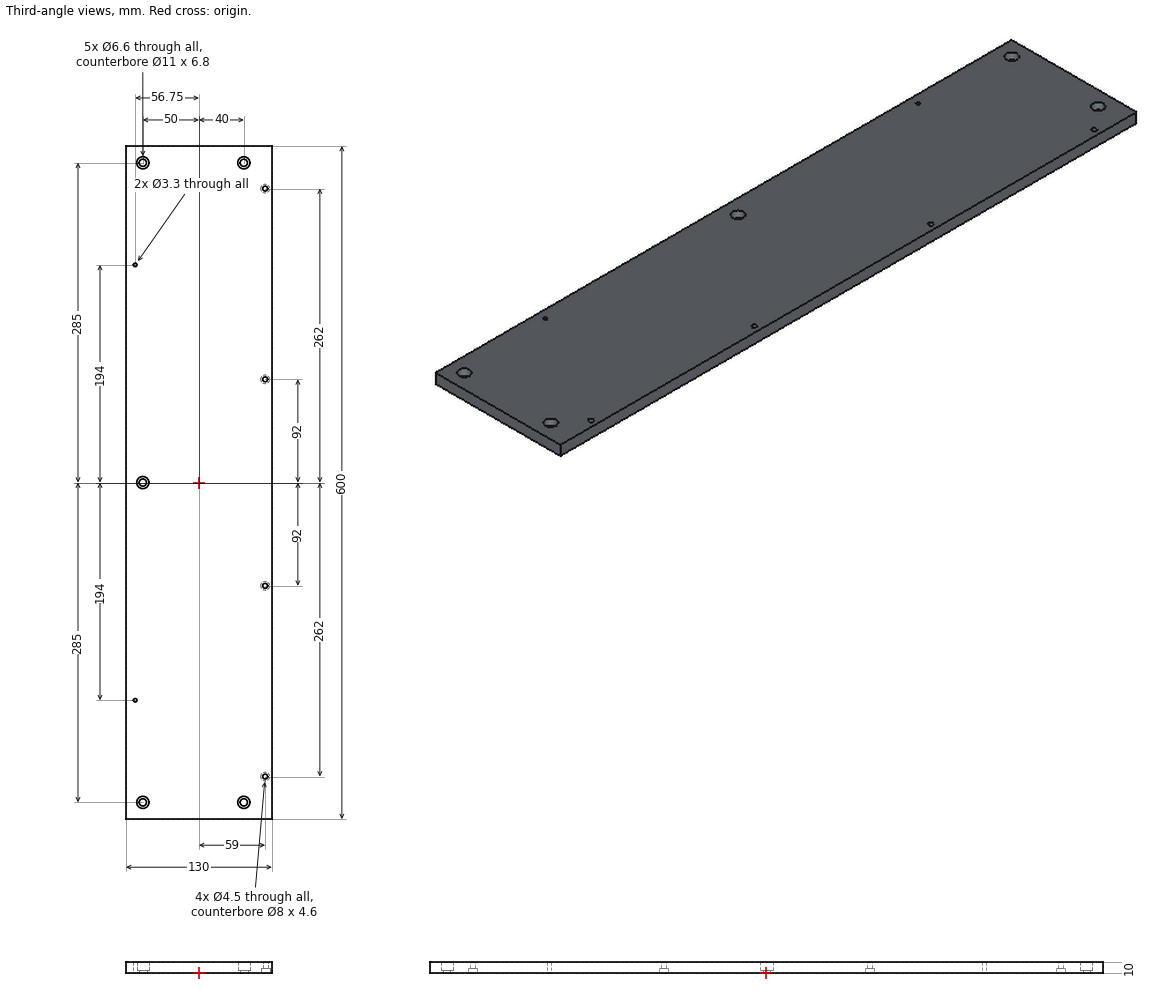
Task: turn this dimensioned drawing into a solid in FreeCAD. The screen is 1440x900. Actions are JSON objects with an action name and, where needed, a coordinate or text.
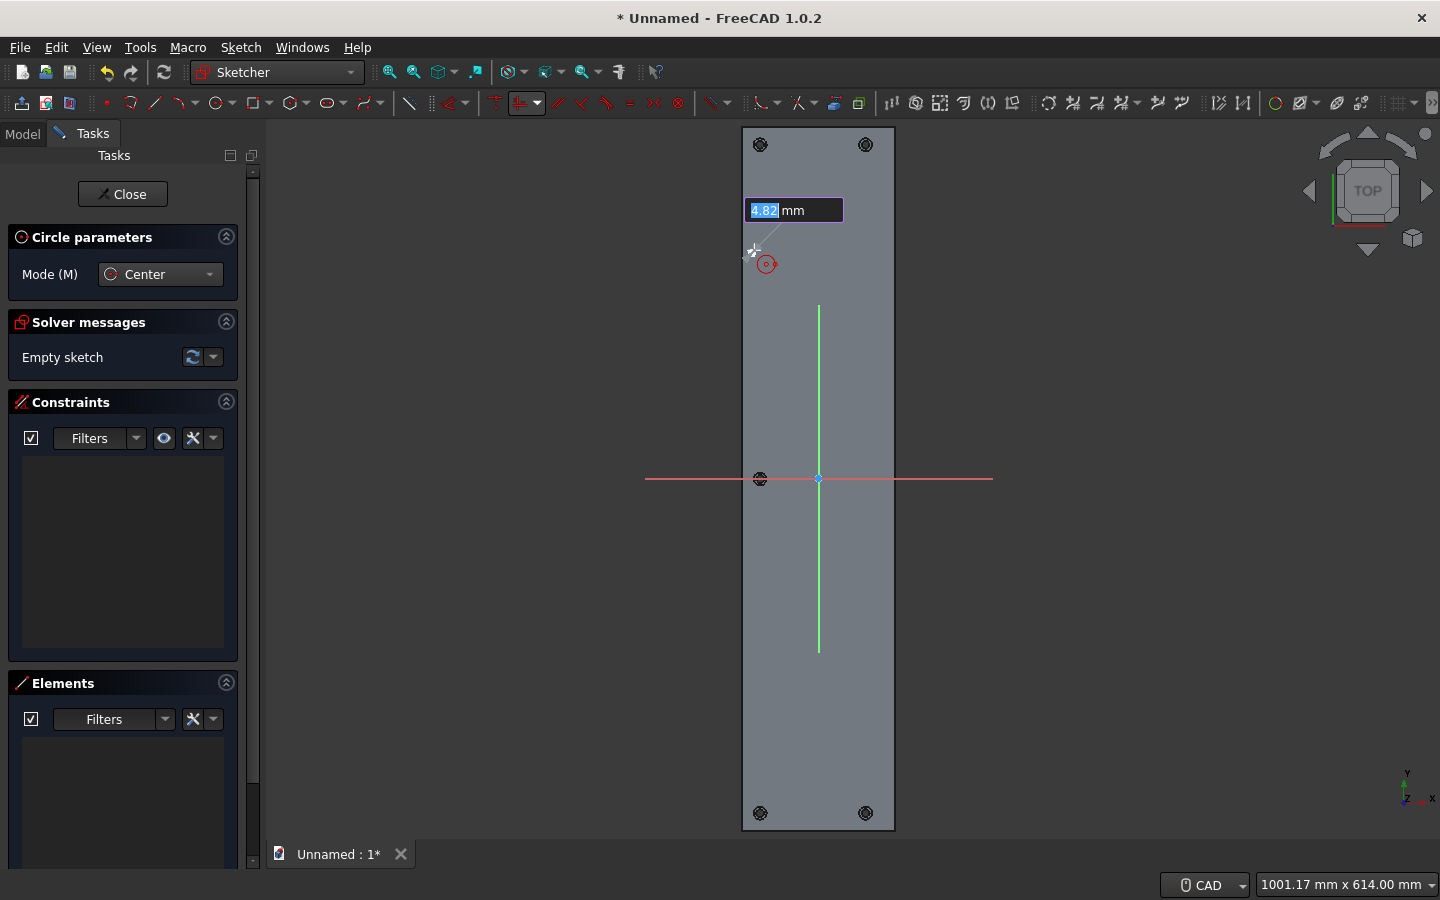
{"action": "type", "text": "3.3"}
{"action": "key", "text": "Return"}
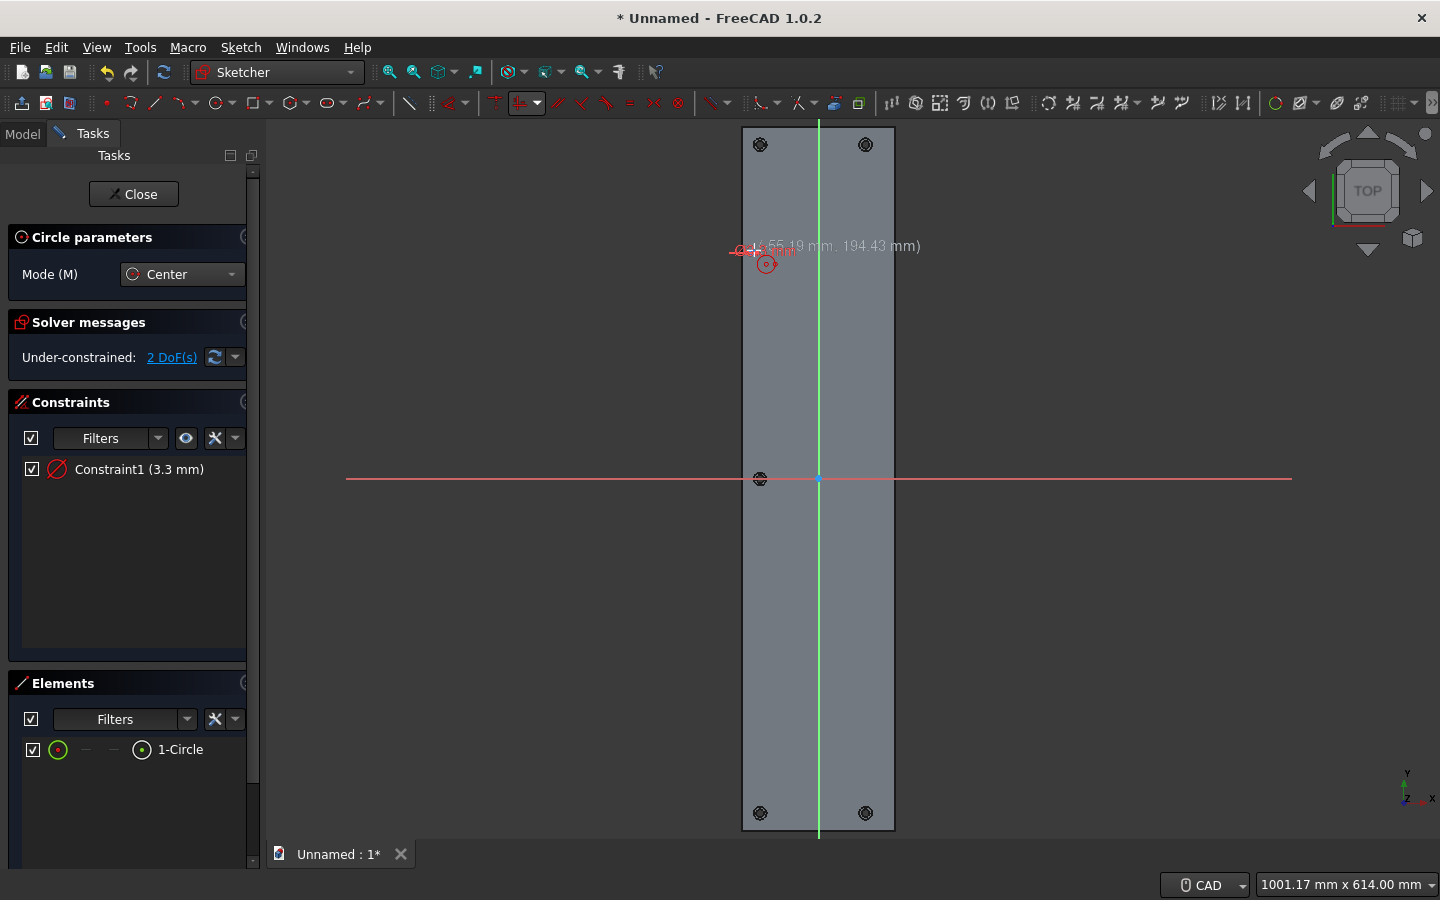
{"action": "scroll", "coordinate": [752, 706], "scroll_direction": "up", "scroll_amount": 13}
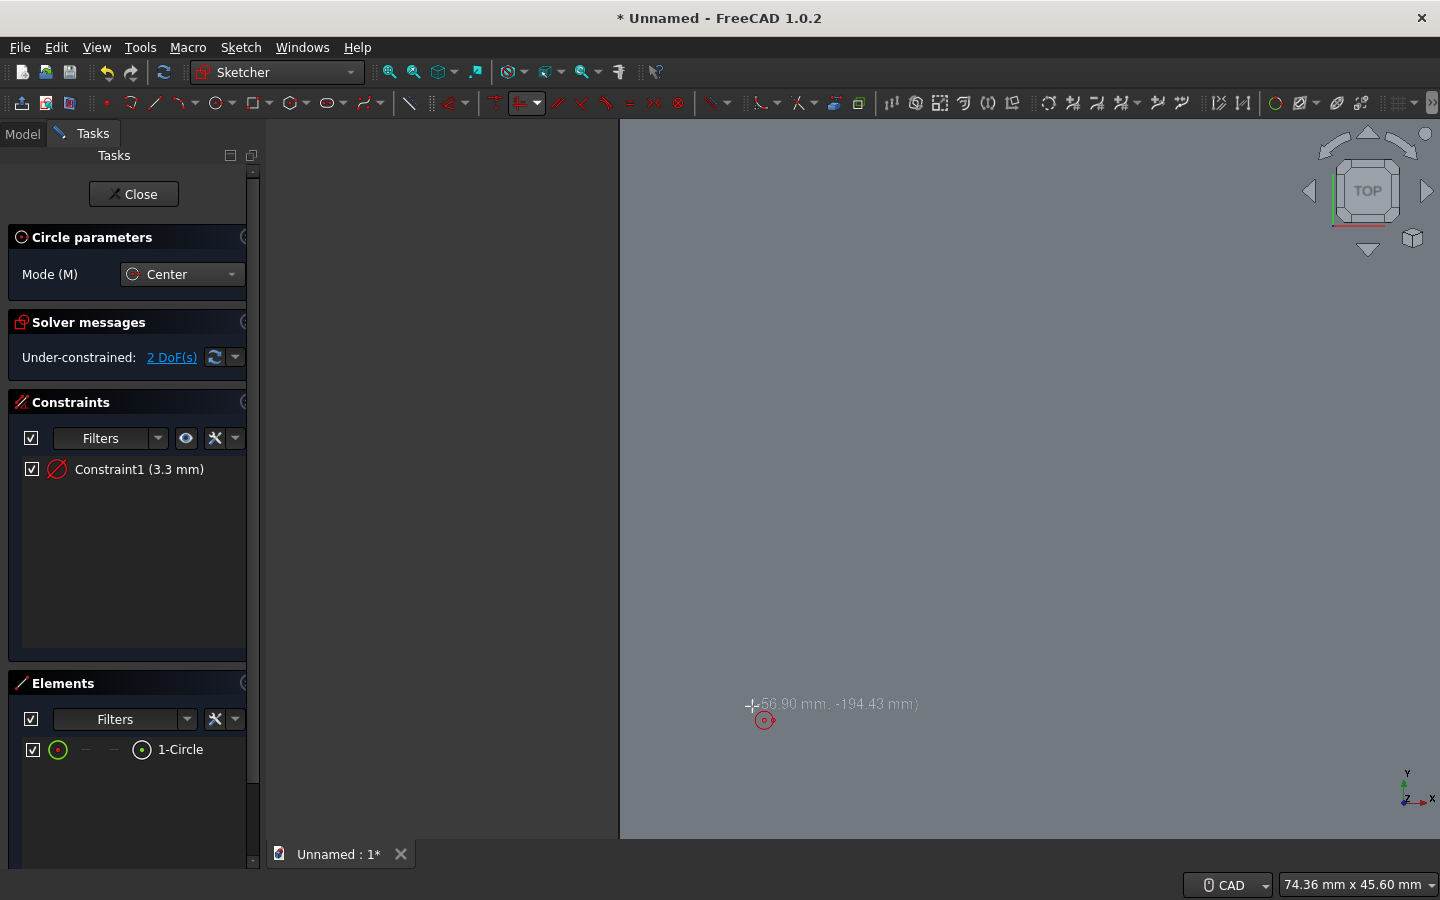
{"action": "scroll", "coordinate": [752, 707], "scroll_direction": "down", "scroll_amount": 13}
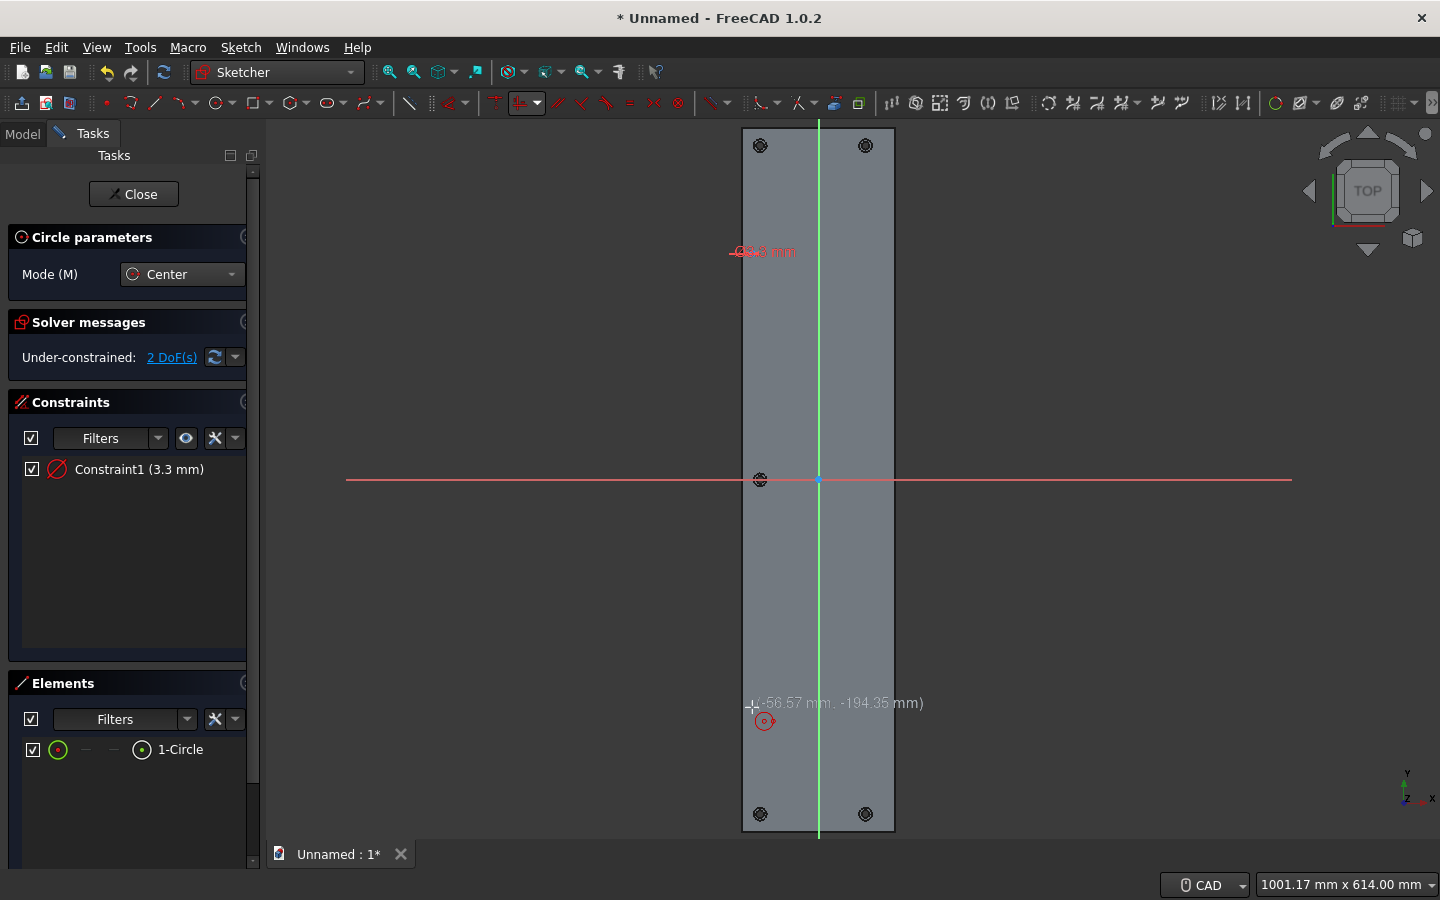
{"action": "left_click", "coordinate": [752, 707]}
{"action": "mouse_move", "coordinate": [754, 706]}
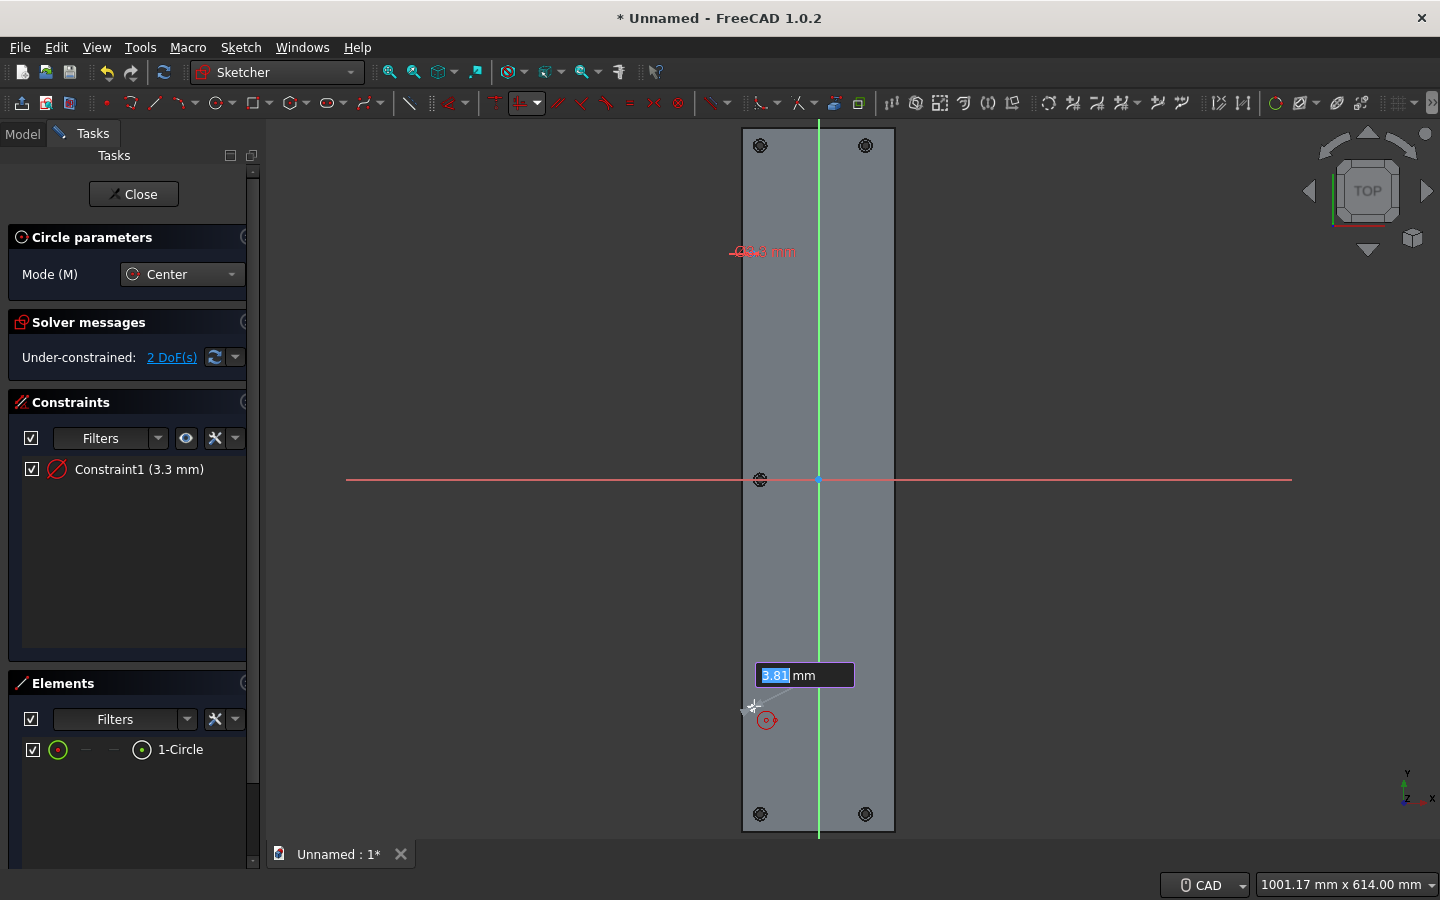
{"action": "type", "text": "3.3"}
{"action": "key", "text": "Return"}
{"action": "key", "text": "Escape"}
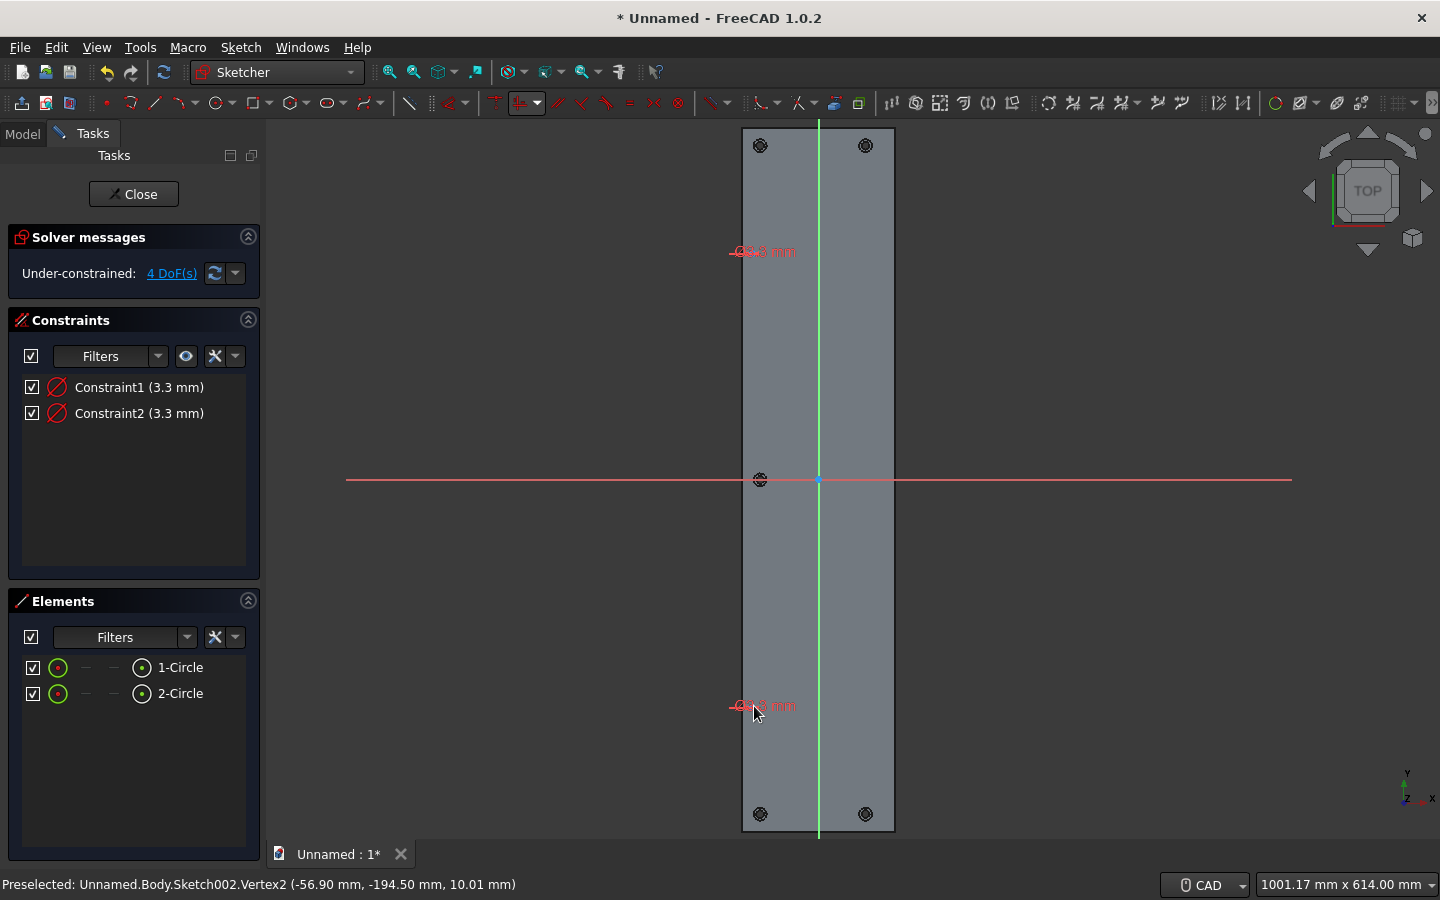
{"action": "left_click", "coordinate": [752, 254]}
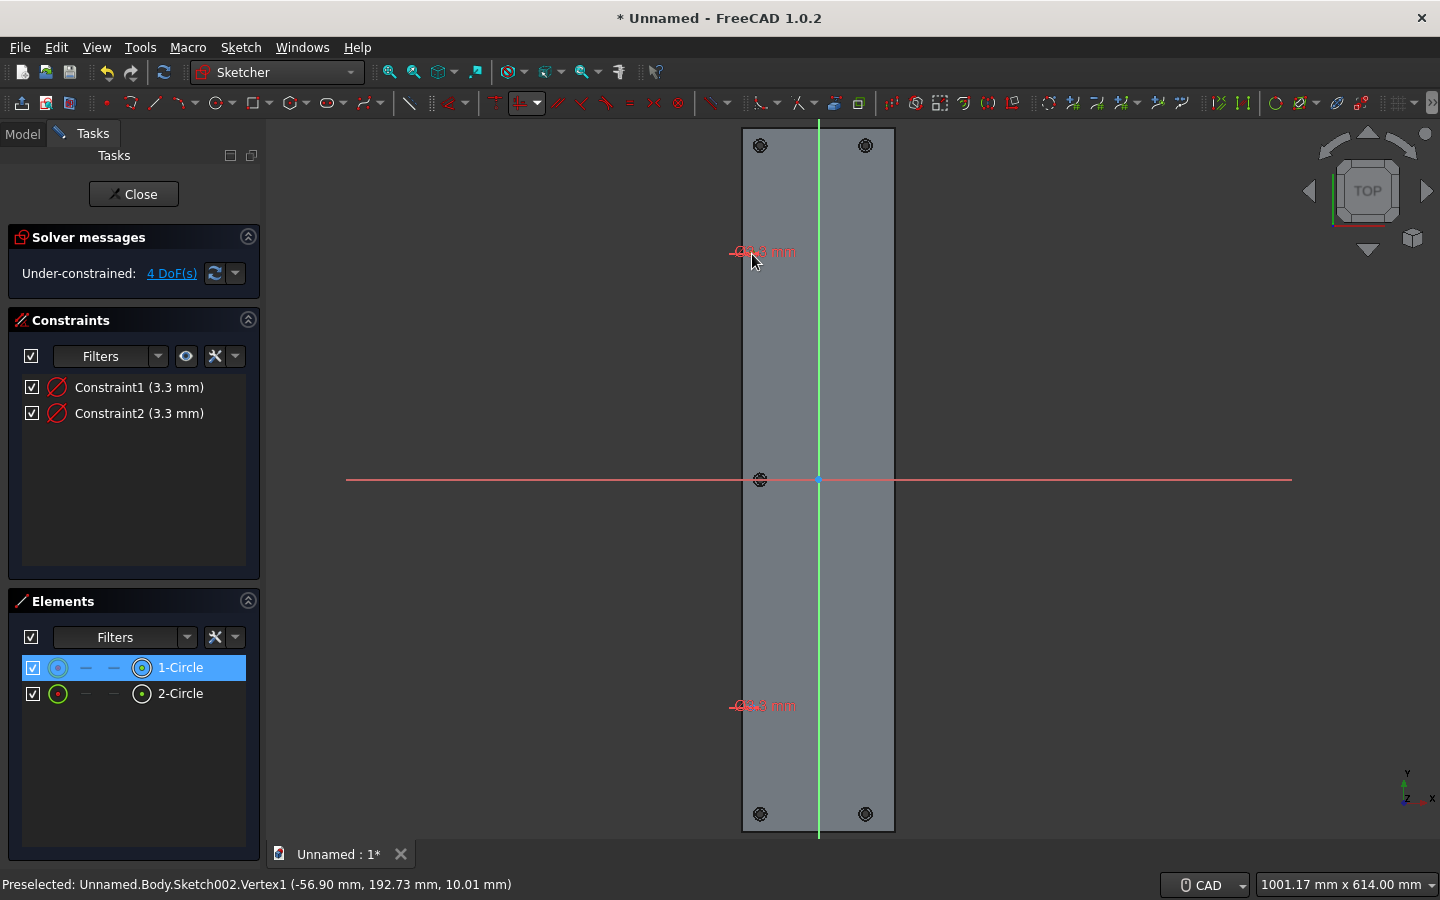
{"action": "left_click", "coordinate": [752, 708]}